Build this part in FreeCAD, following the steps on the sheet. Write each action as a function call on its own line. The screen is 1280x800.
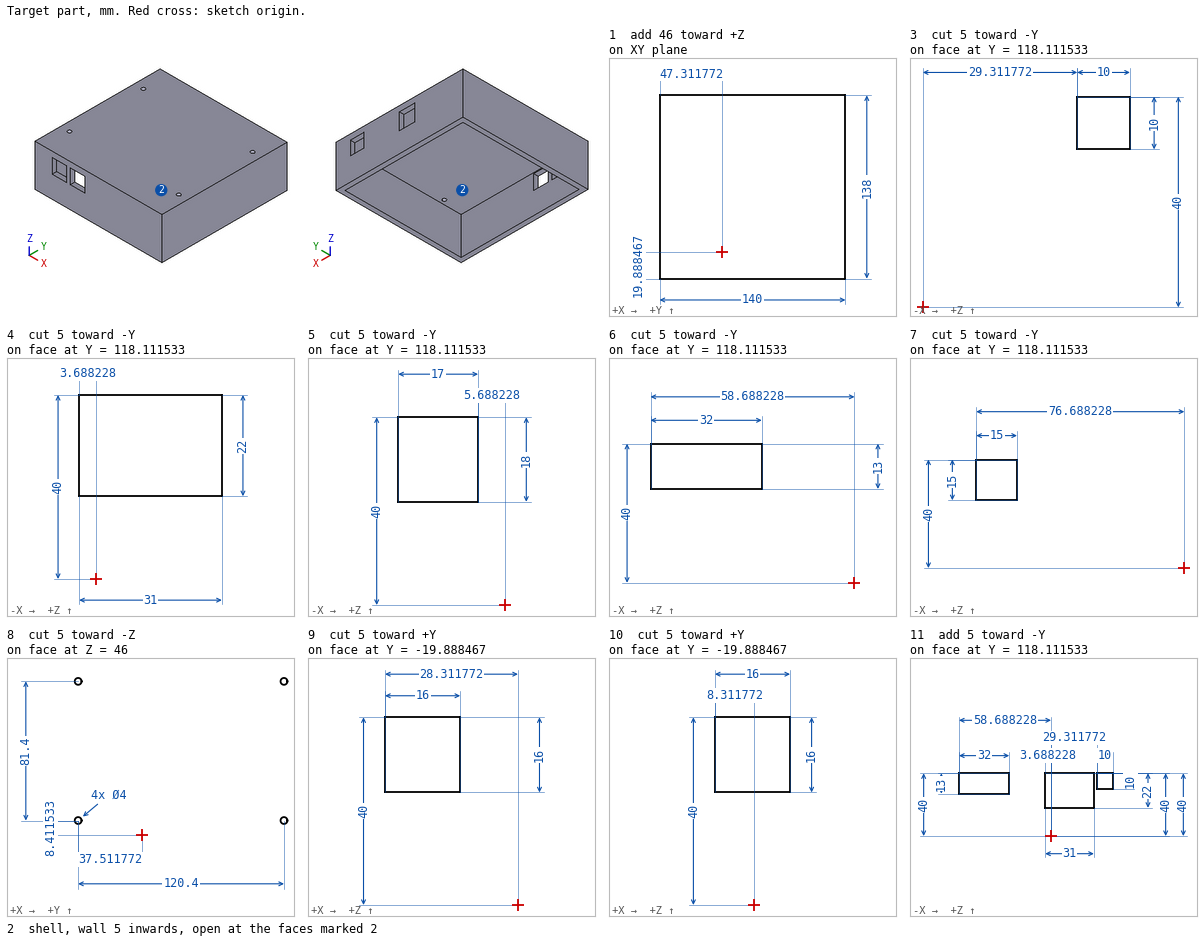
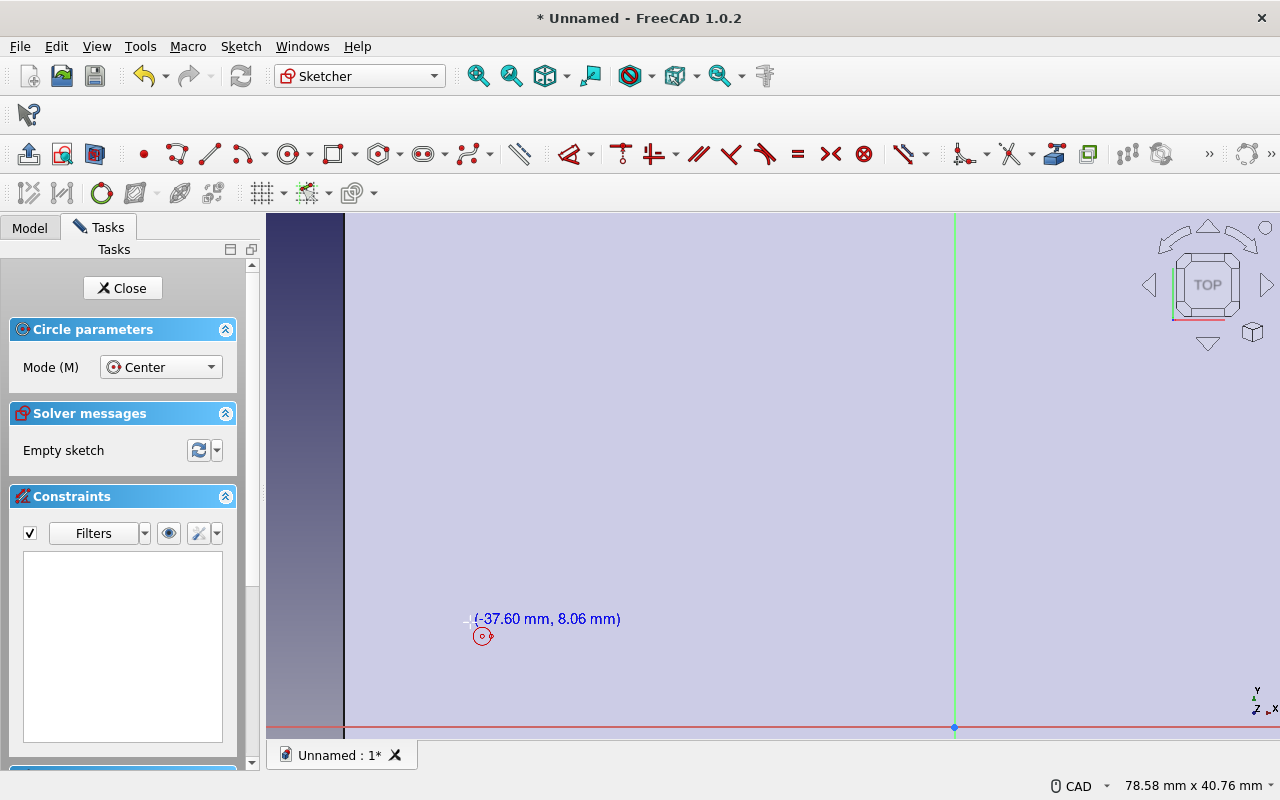
click(471, 619)
move(489, 601)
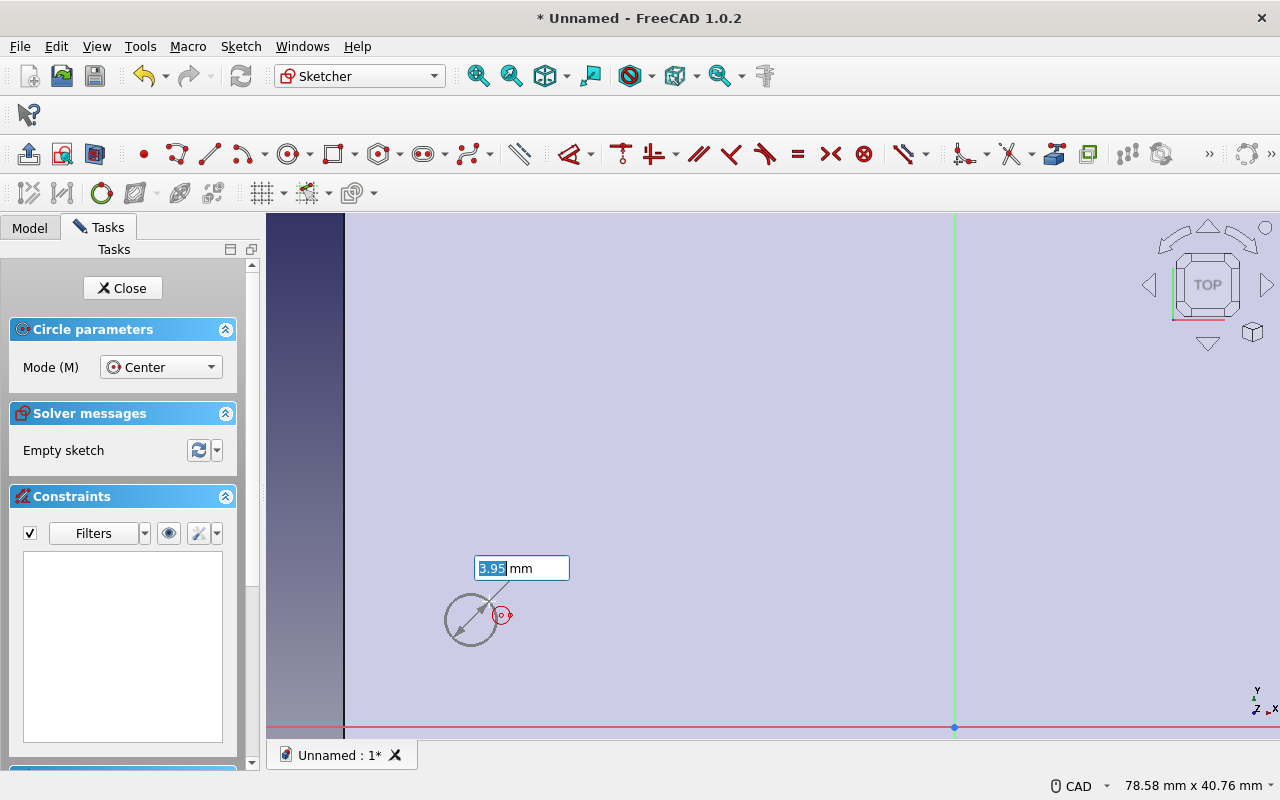
text(4)
key(Return)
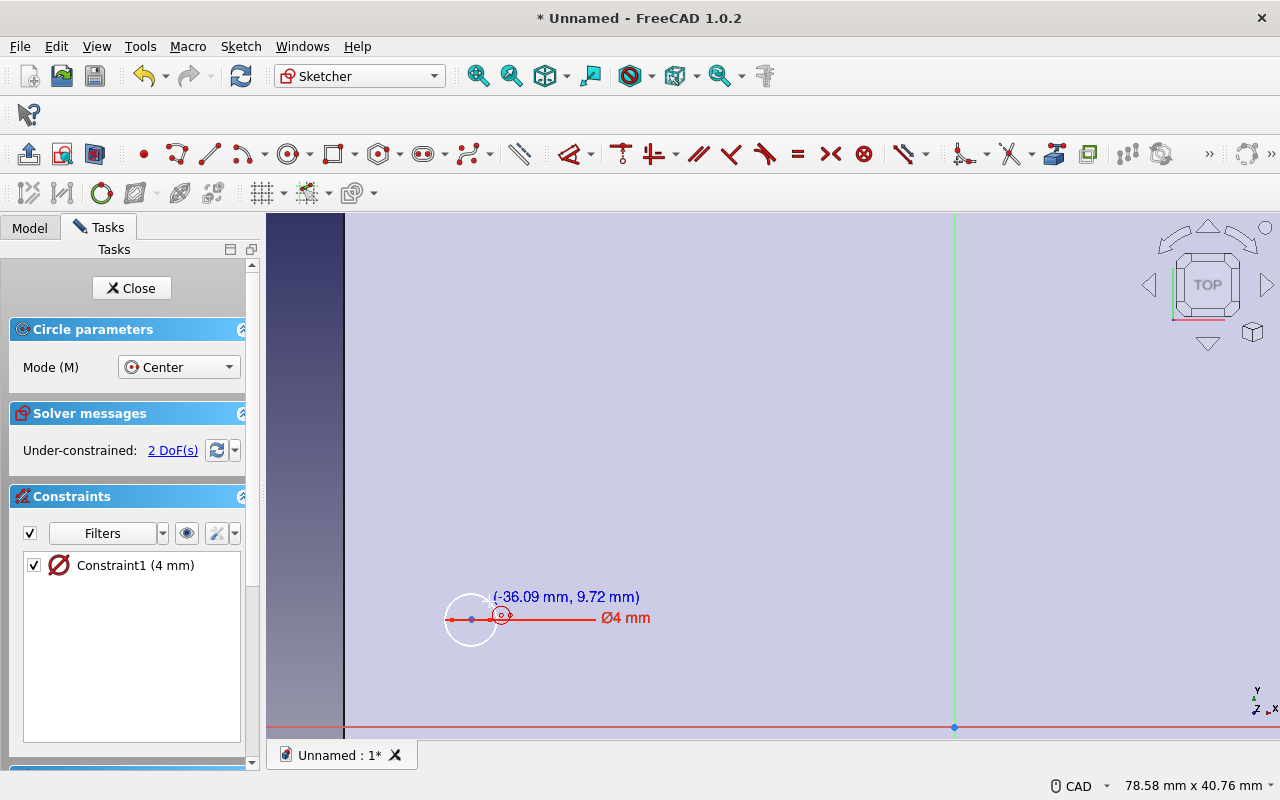
scroll(470, 623, down, 6)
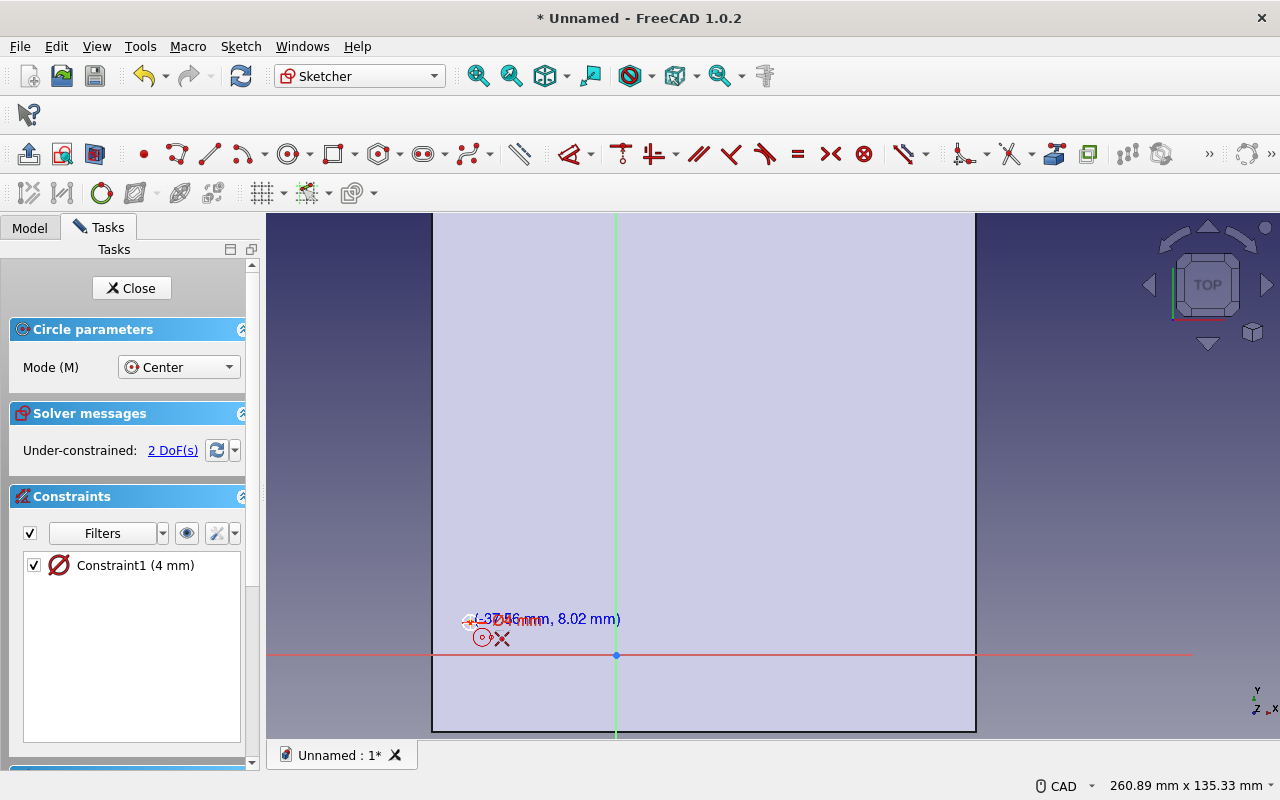
scroll(470, 306, up, 6)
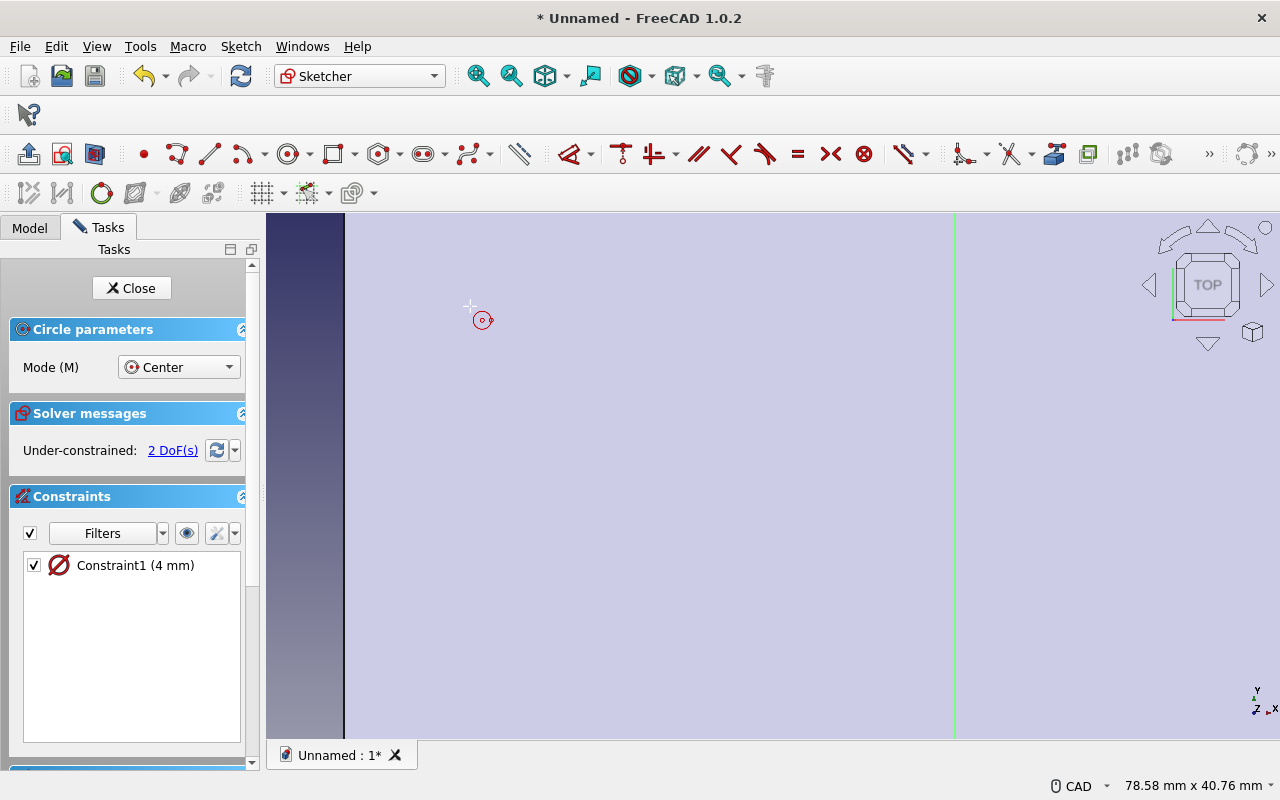
click(471, 305)
move(489, 287)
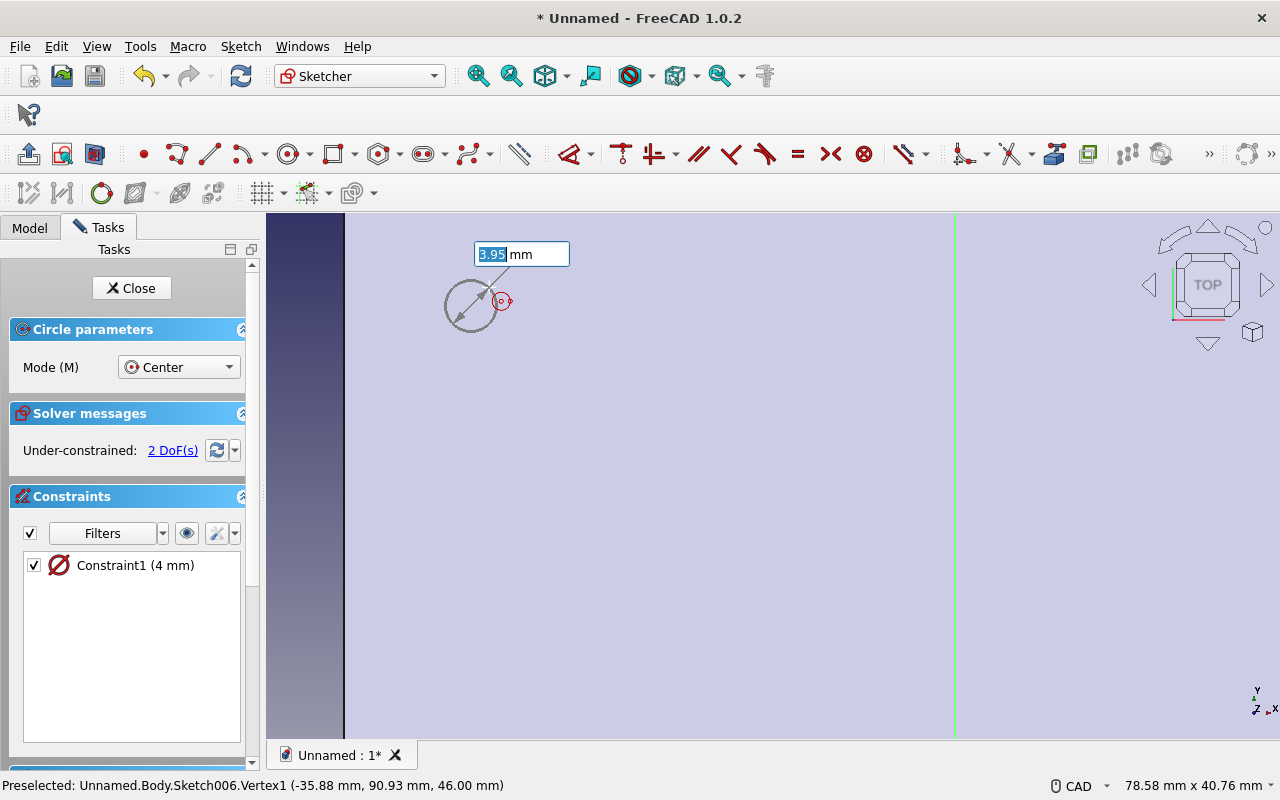
text(4)
key(Return)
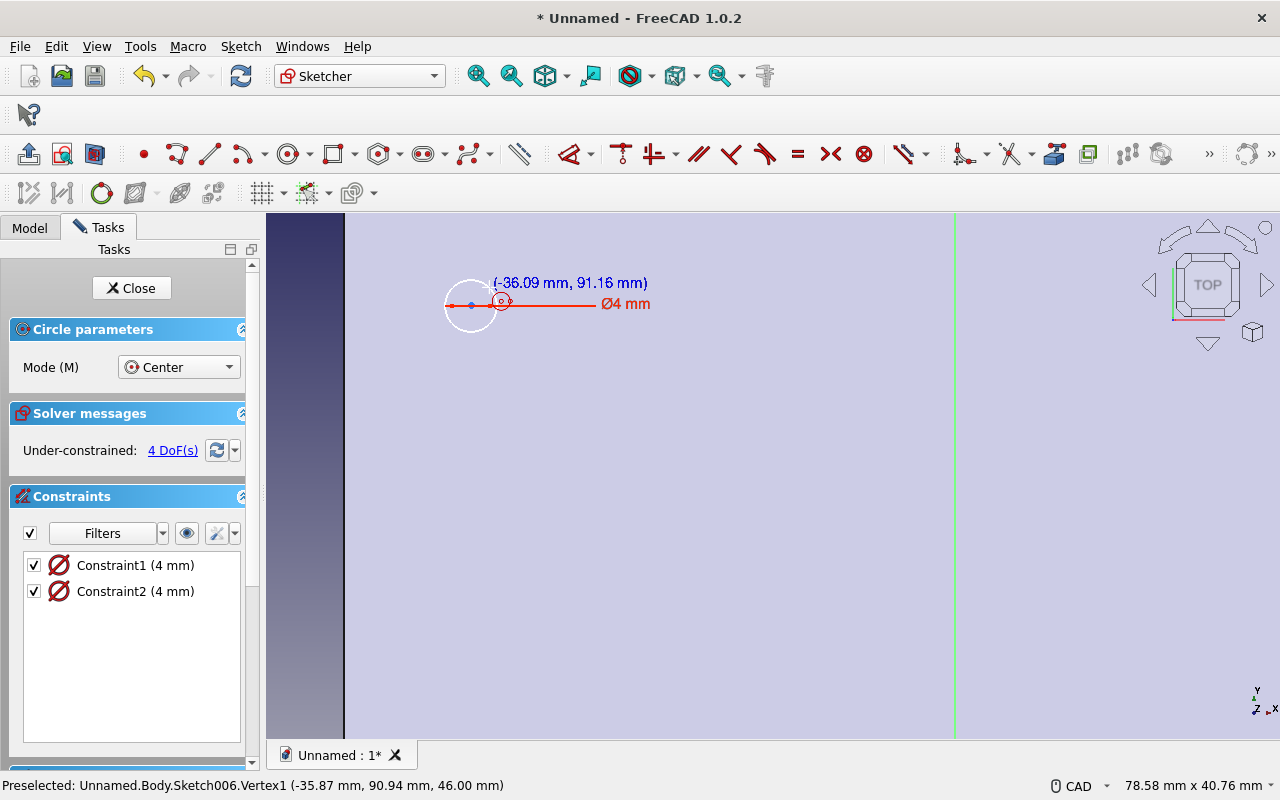
scroll(470, 305, down, 6)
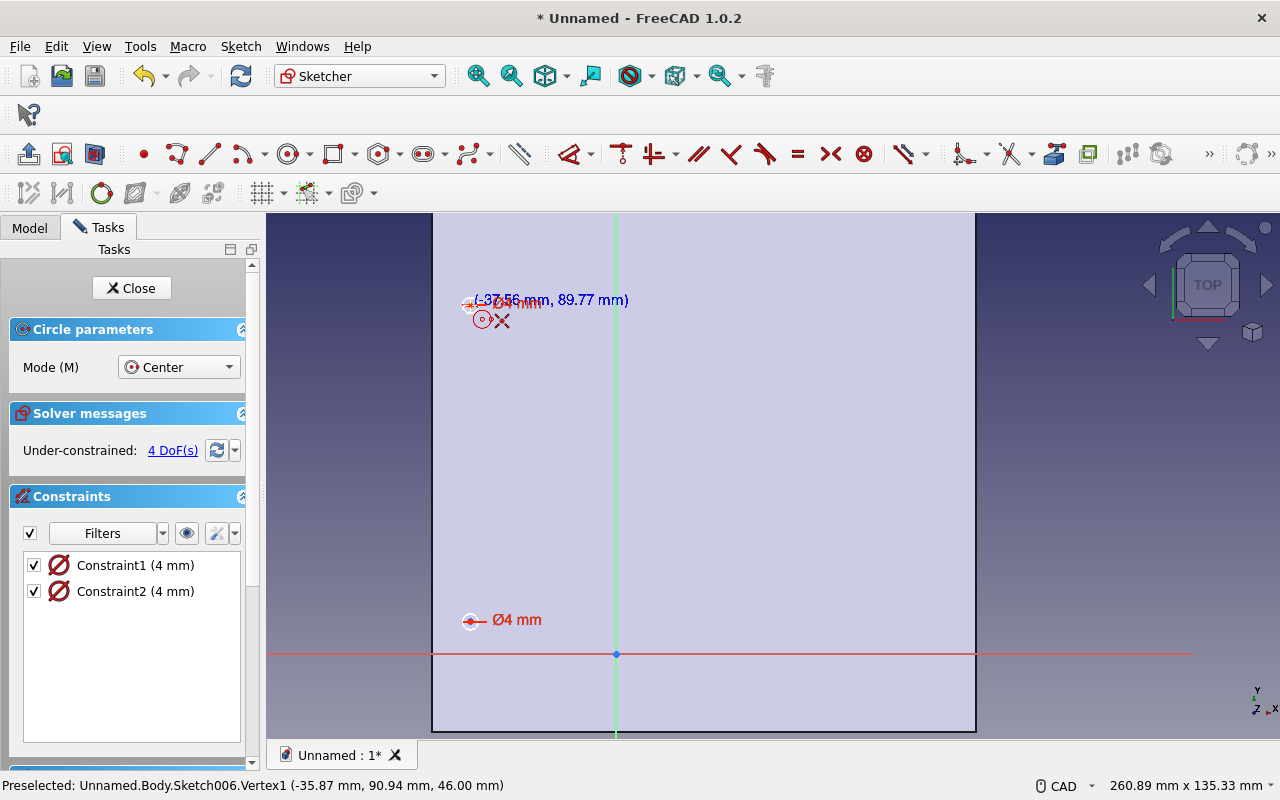
scroll(938, 622, up, 6)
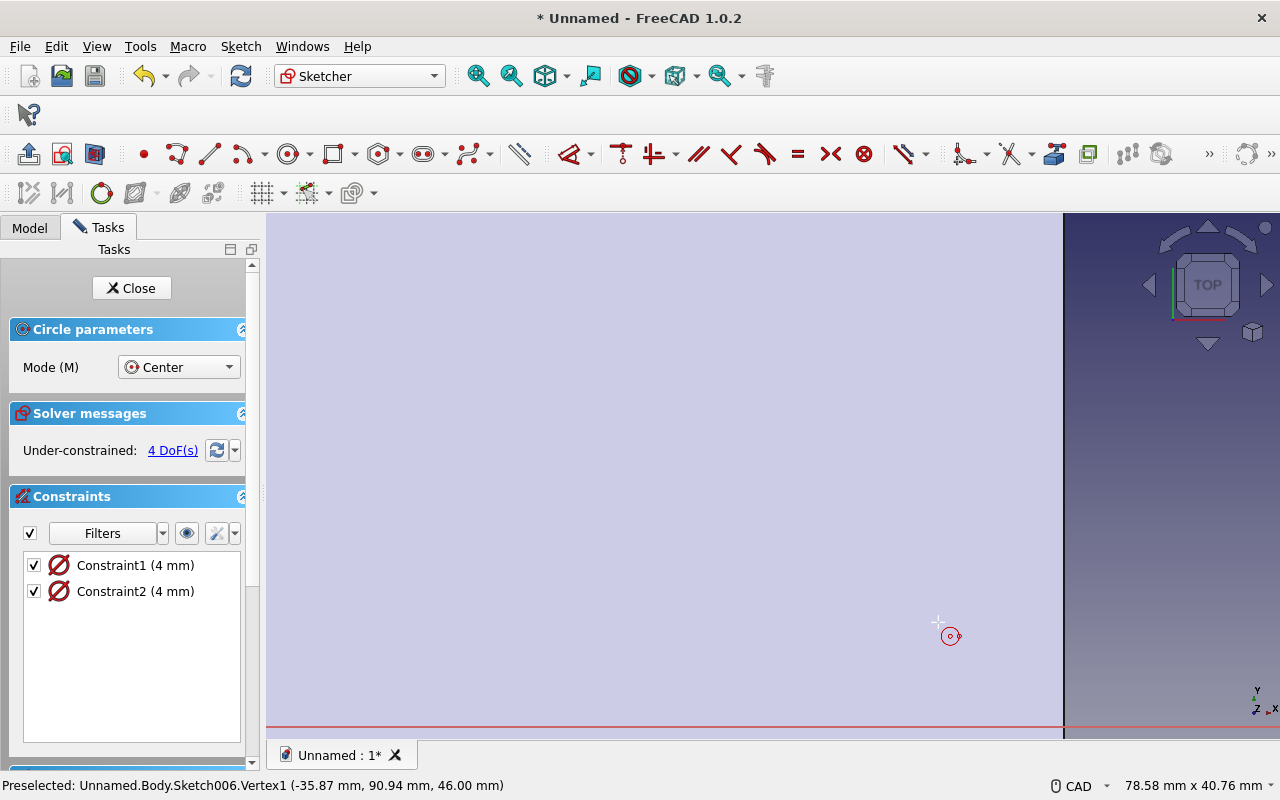
click(937, 619)
move(956, 601)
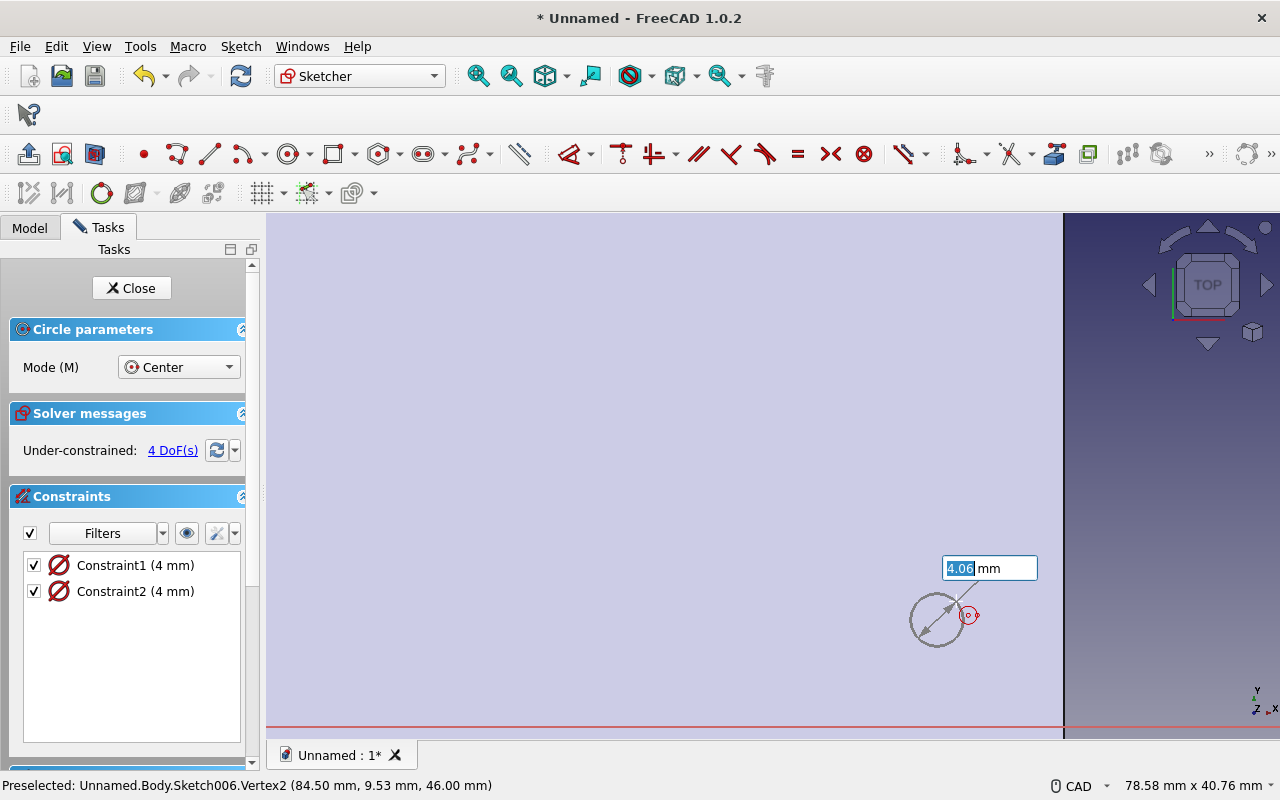
text(4)
key(Return)